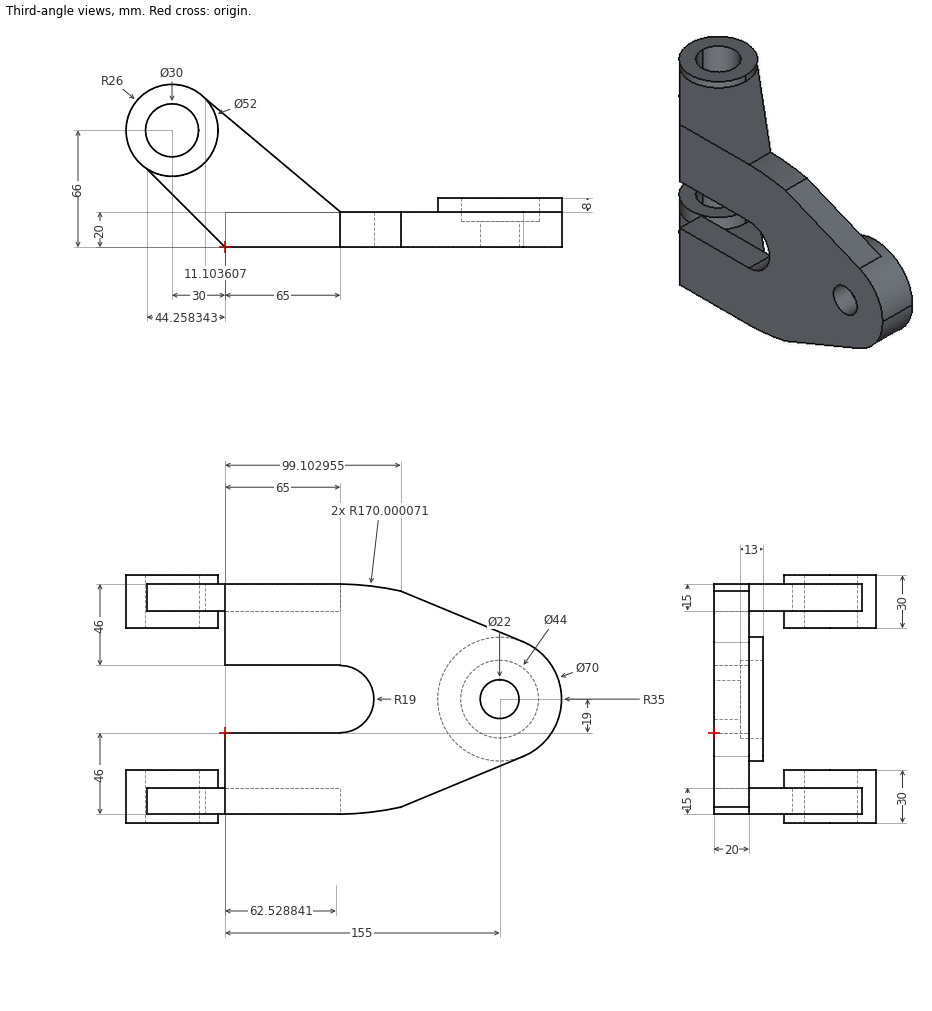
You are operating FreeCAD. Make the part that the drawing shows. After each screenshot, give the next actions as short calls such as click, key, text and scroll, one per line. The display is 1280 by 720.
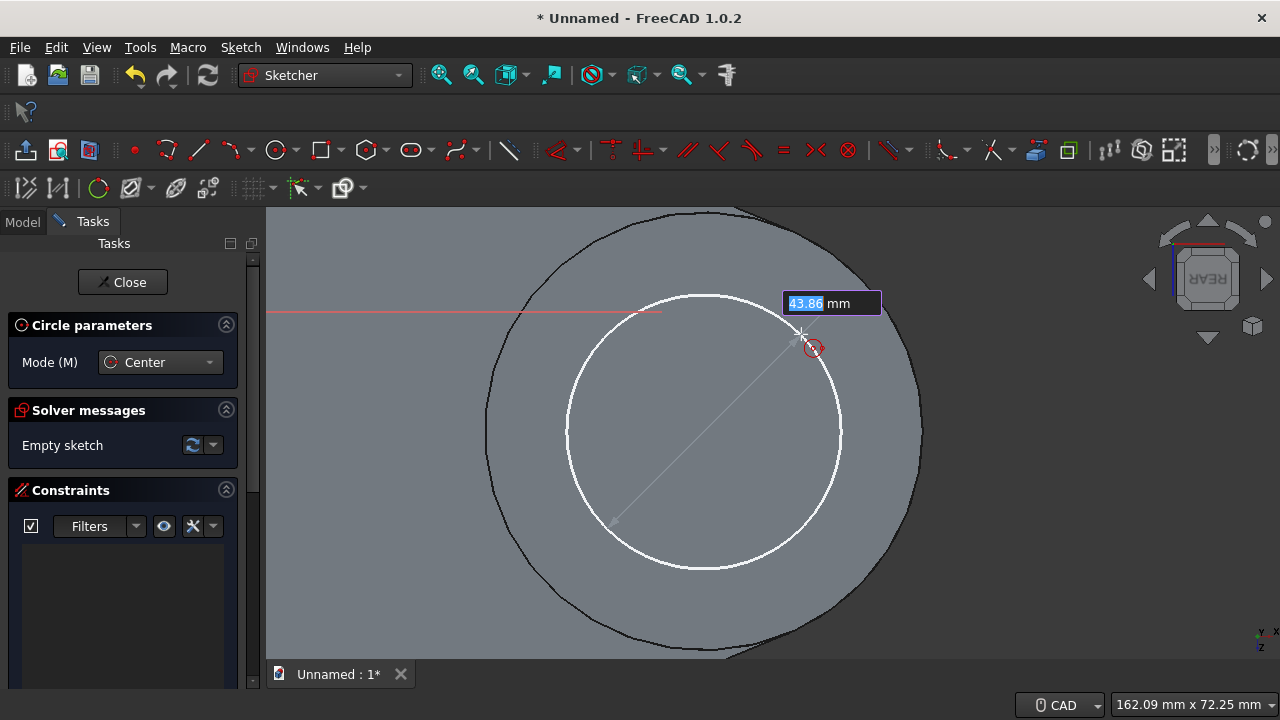
text(44)
key(Return)
key(Escape)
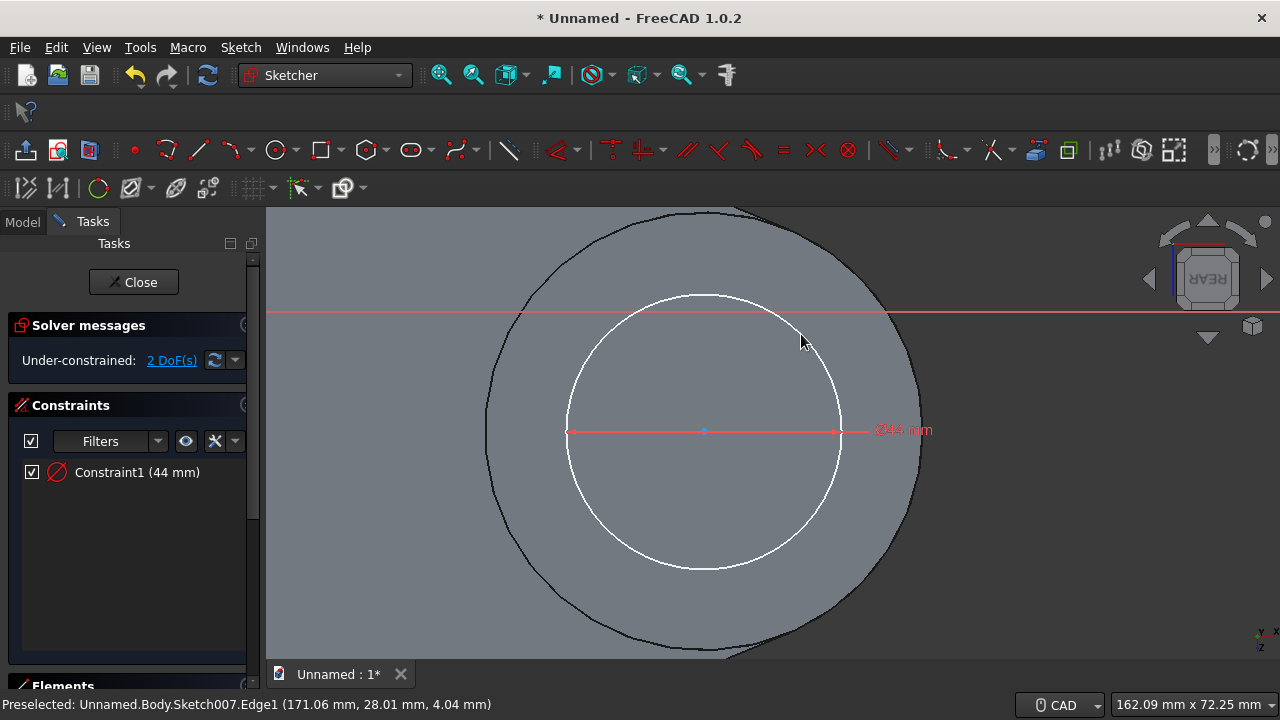
key(d)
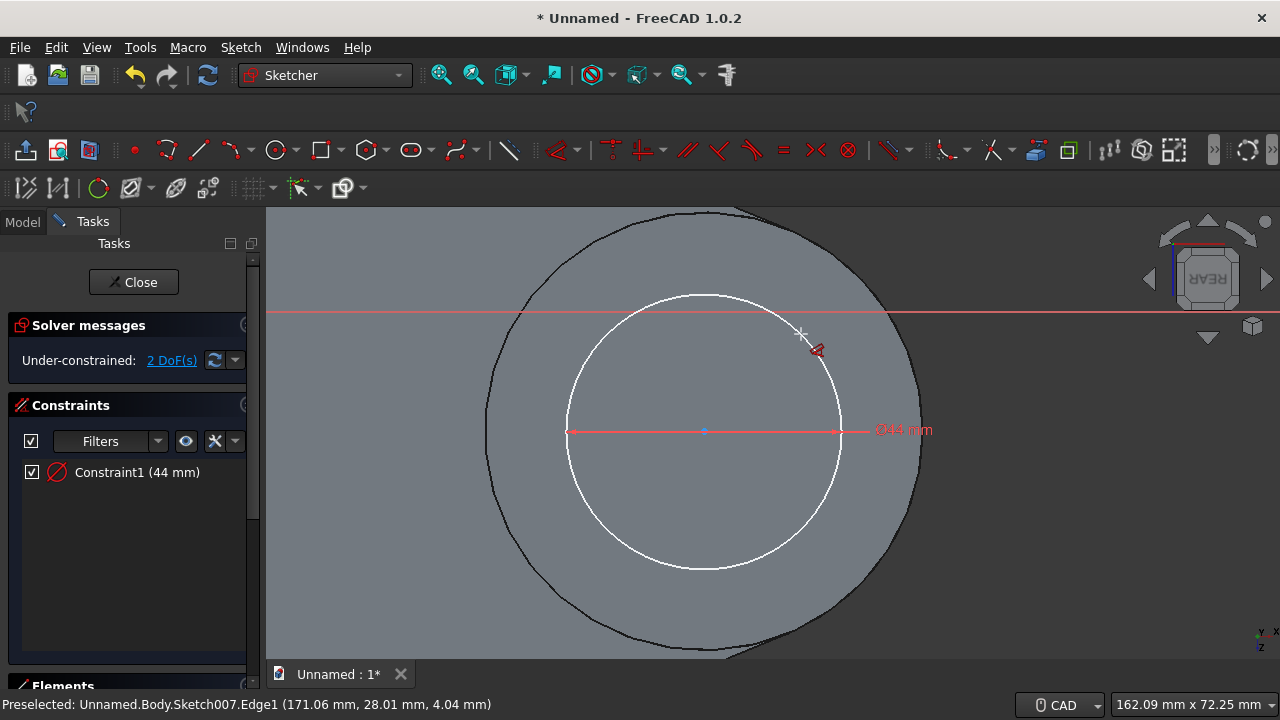
click(704, 432)
click(738, 372)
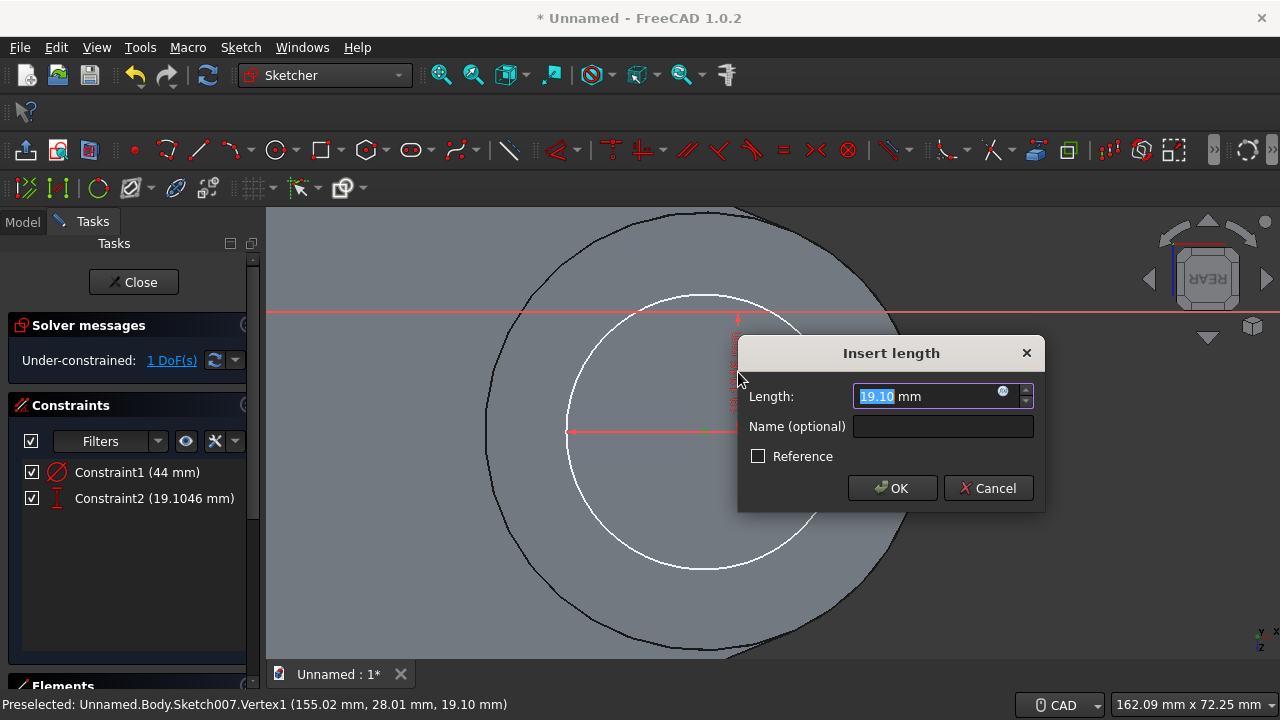
text(19)
key(Return)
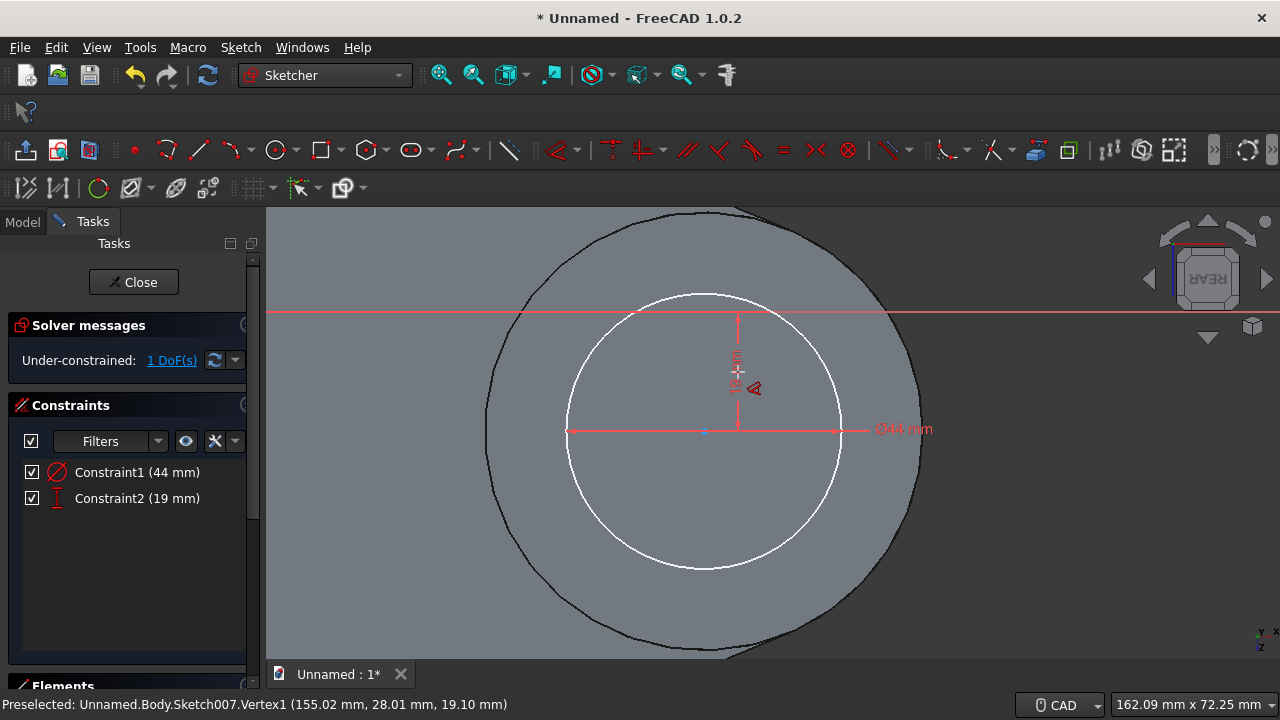
click(704, 431)
click(499, 278)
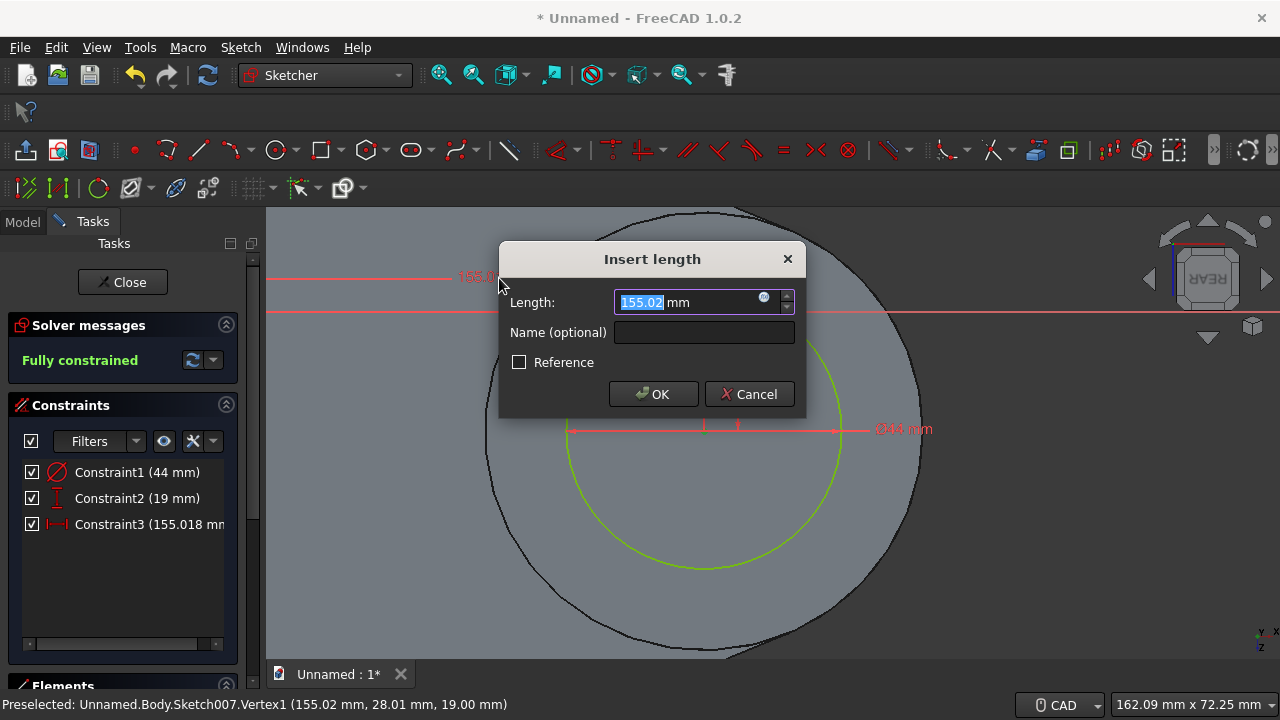
text(155)
key(Return)
key(Escape)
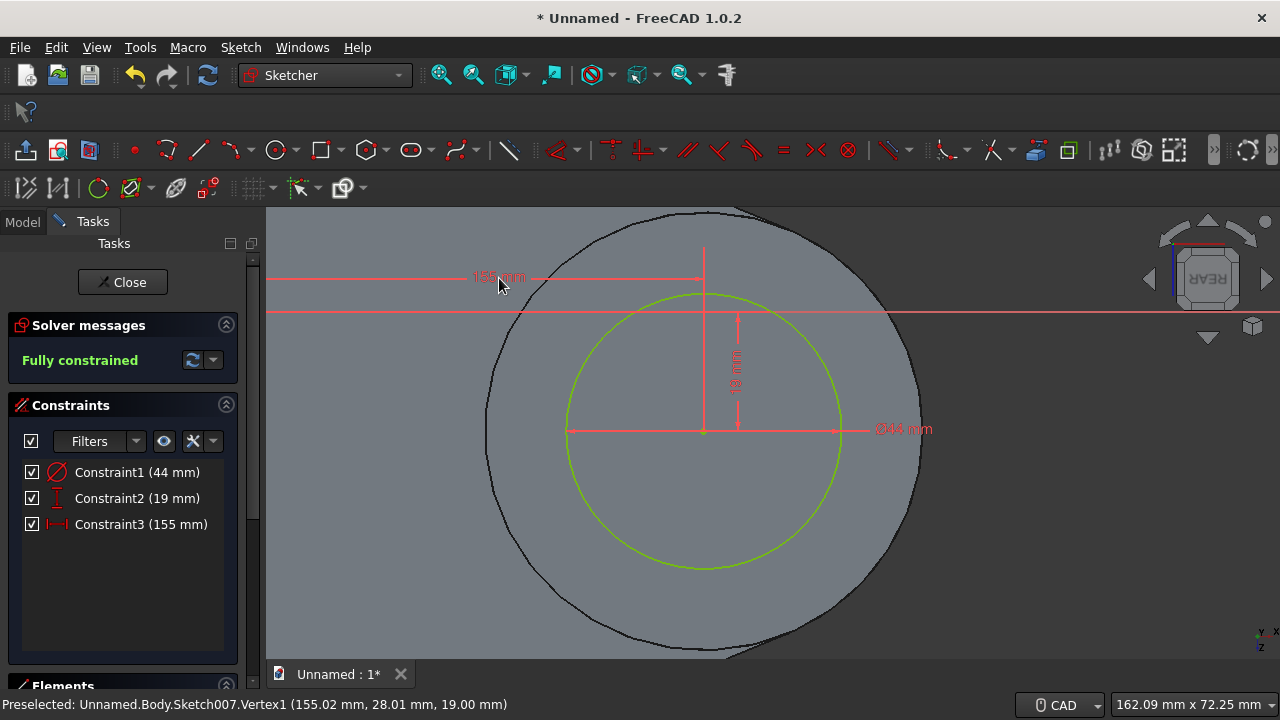
click(123, 282)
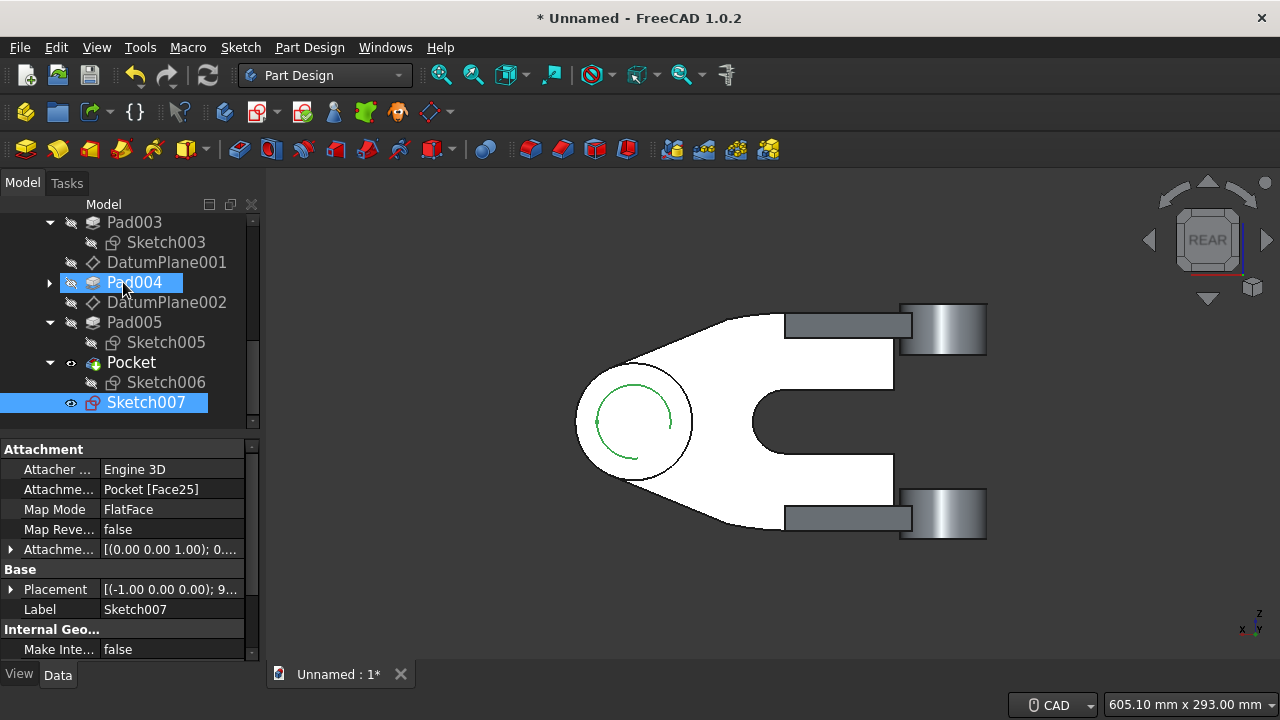
click(240, 150)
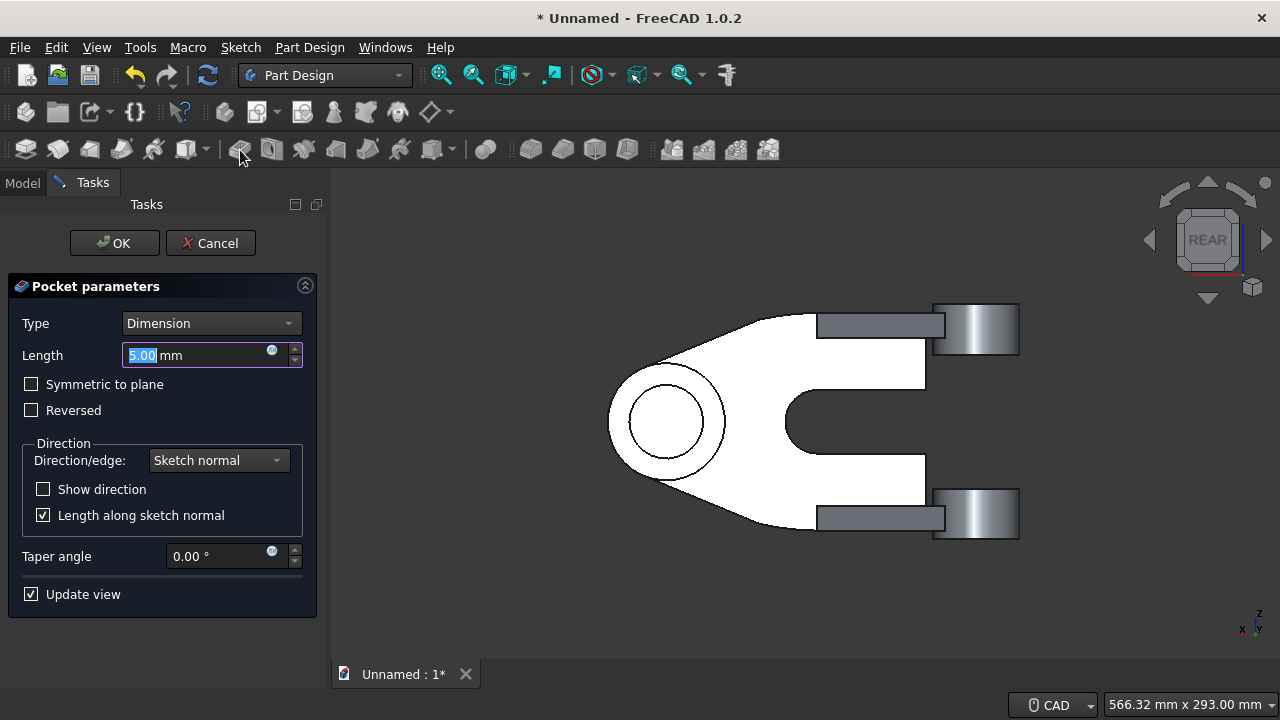
text(13)
key(Tab)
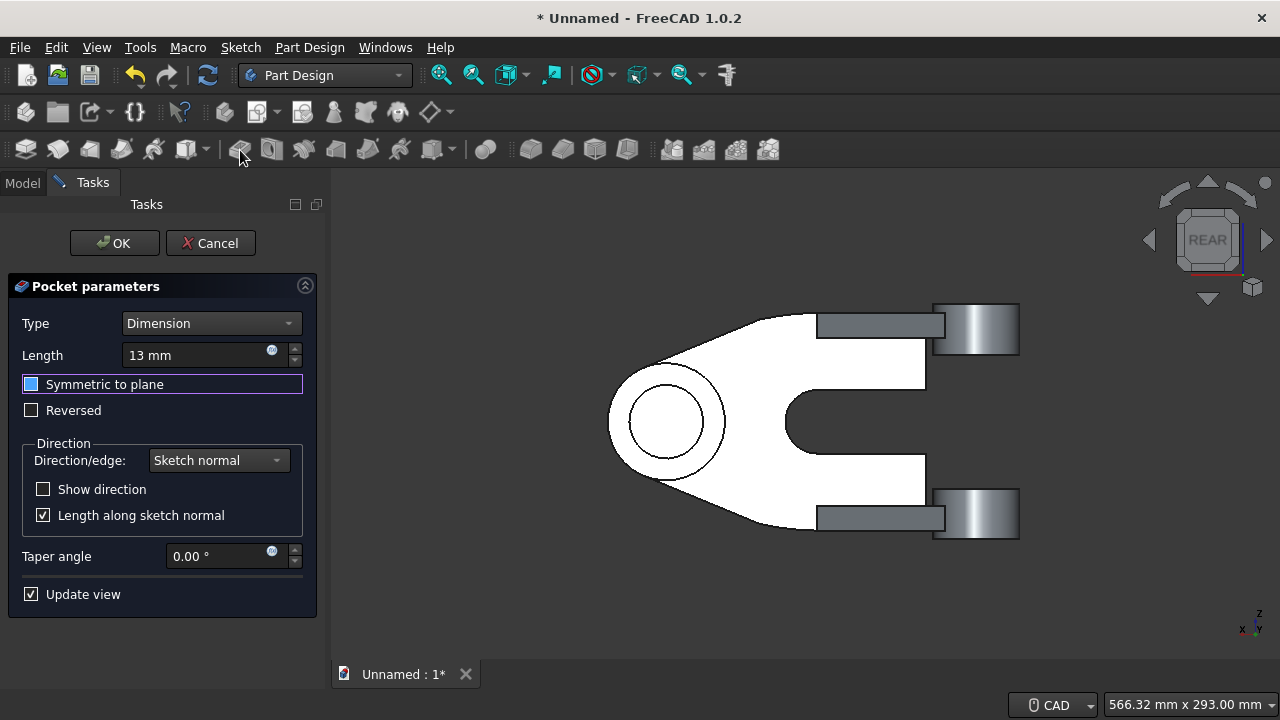
click(115, 243)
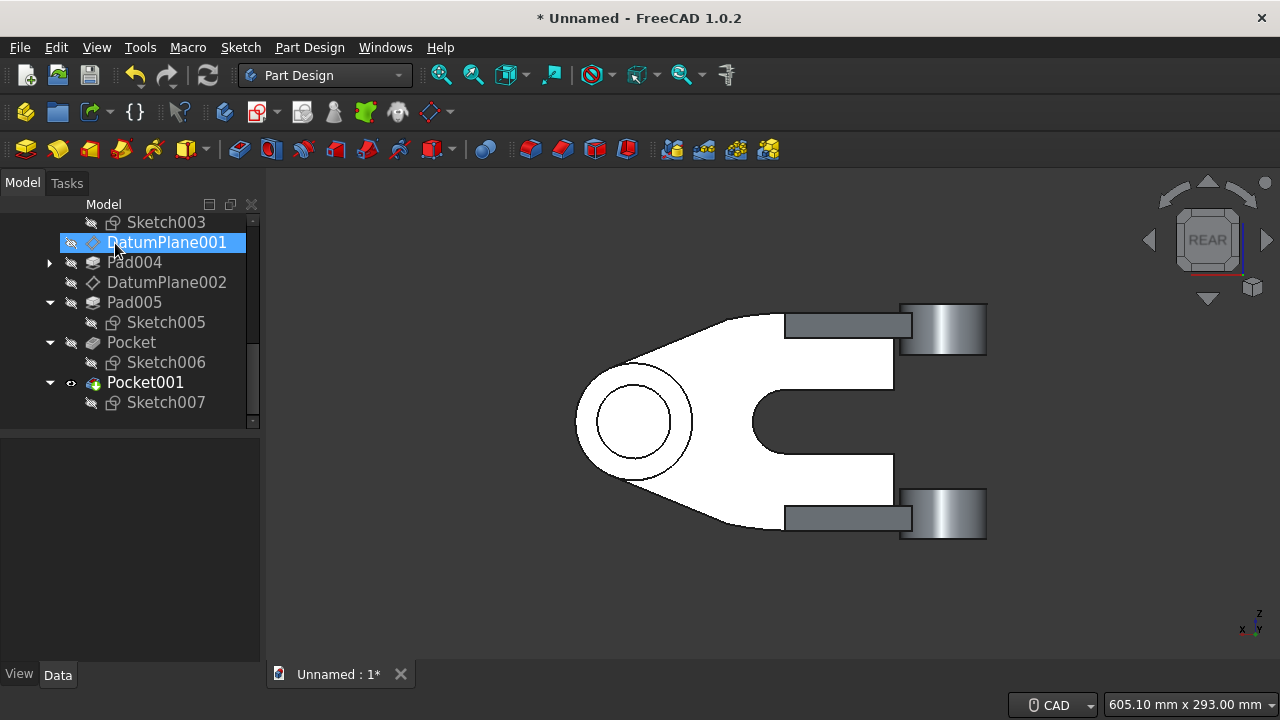
click(634, 421)